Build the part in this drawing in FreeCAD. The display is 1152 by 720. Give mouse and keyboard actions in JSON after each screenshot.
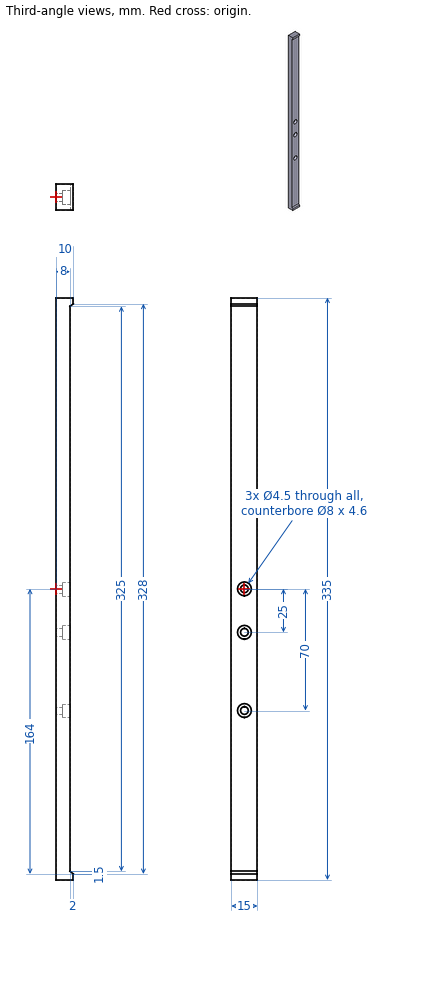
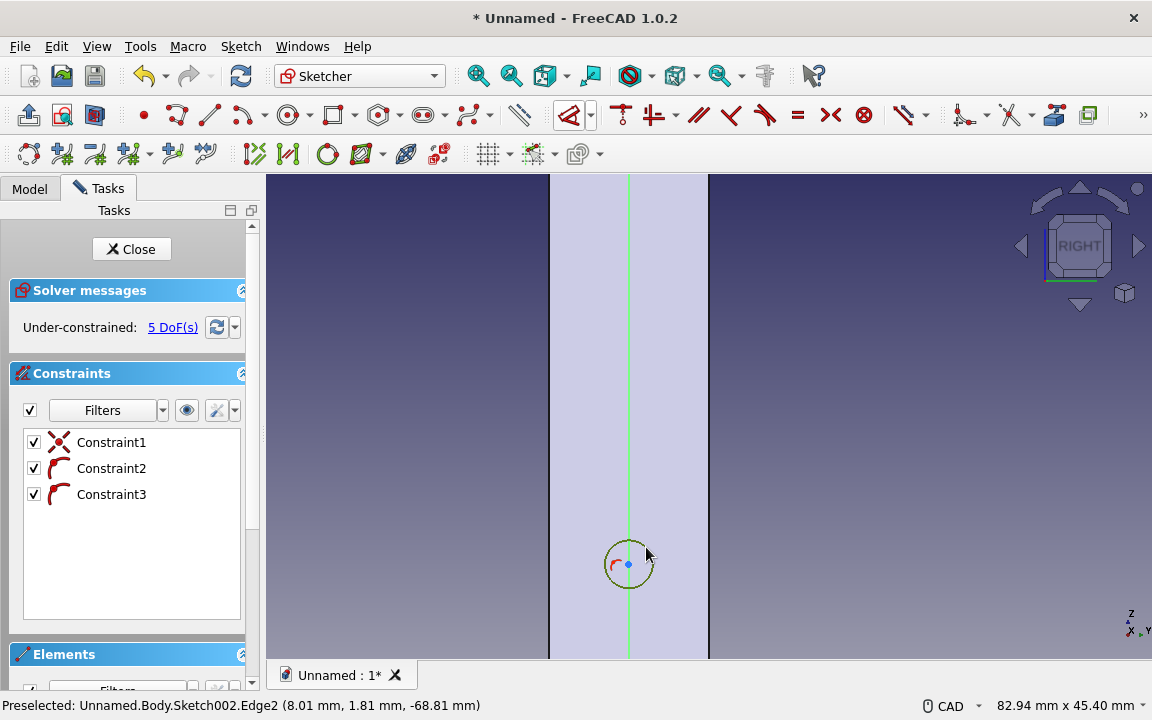
{"action": "scroll", "coordinate": [647, 549], "scroll_direction": "down", "scroll_amount": 5}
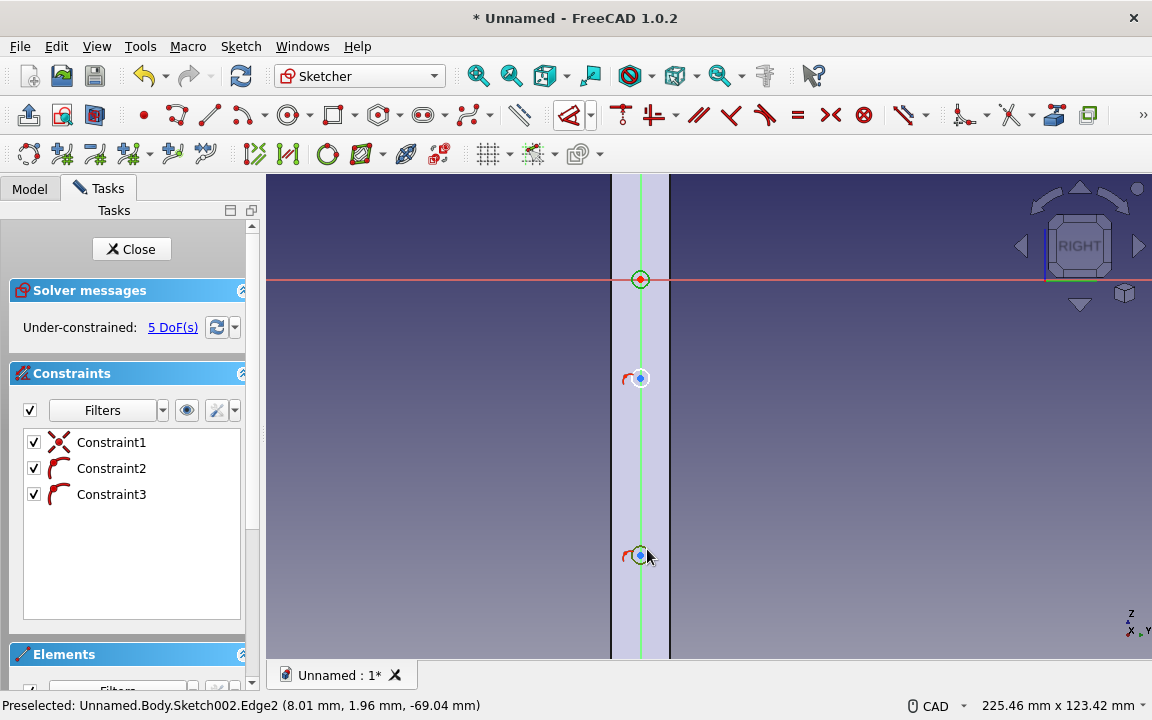
{"action": "scroll", "coordinate": [647, 372], "scroll_direction": "up", "scroll_amount": 5}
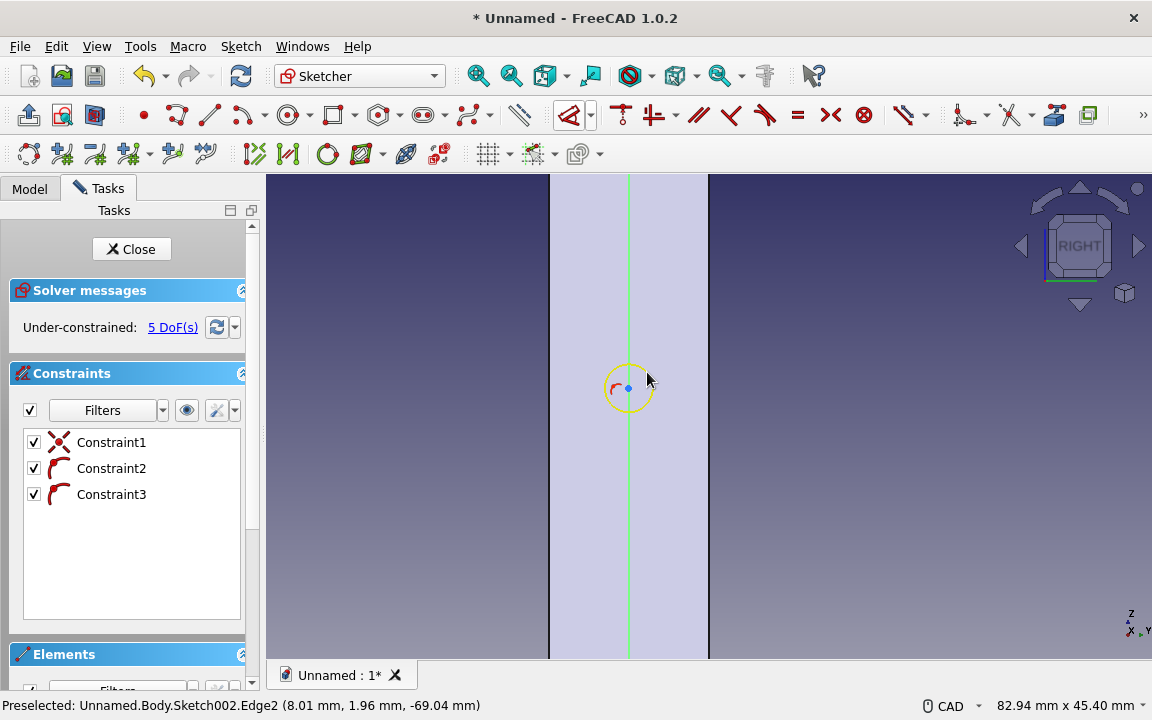
{"action": "left_click", "coordinate": [646, 371]}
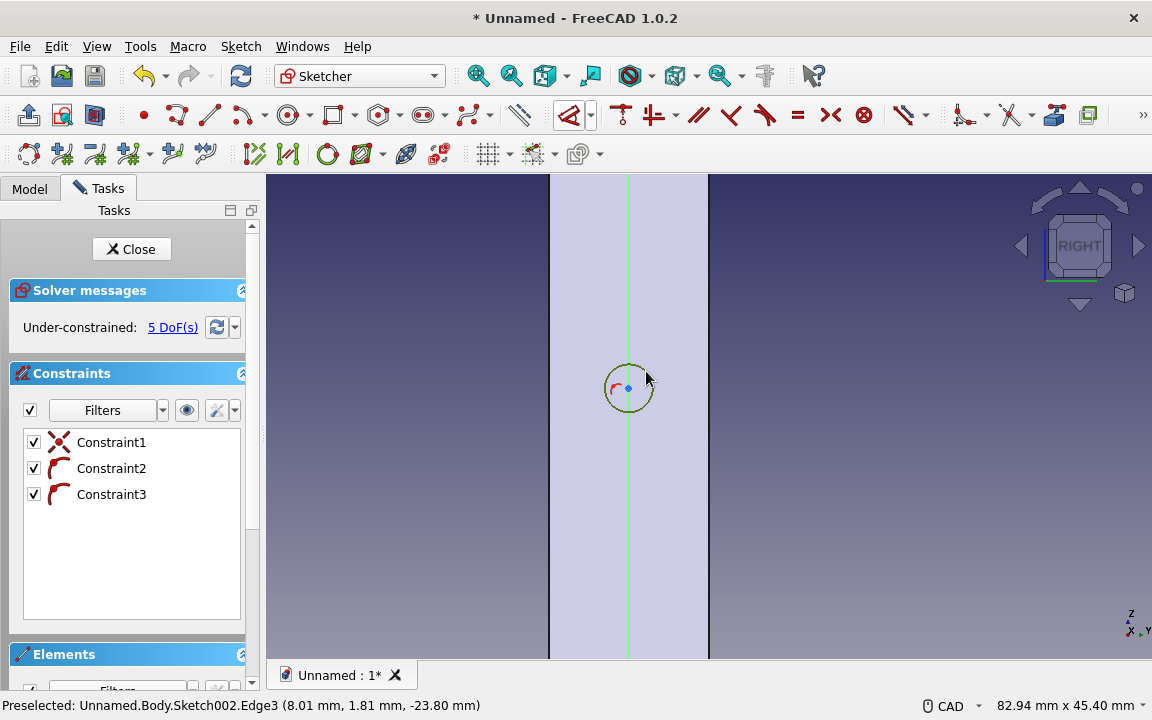
{"action": "left_click", "coordinate": [798, 116]}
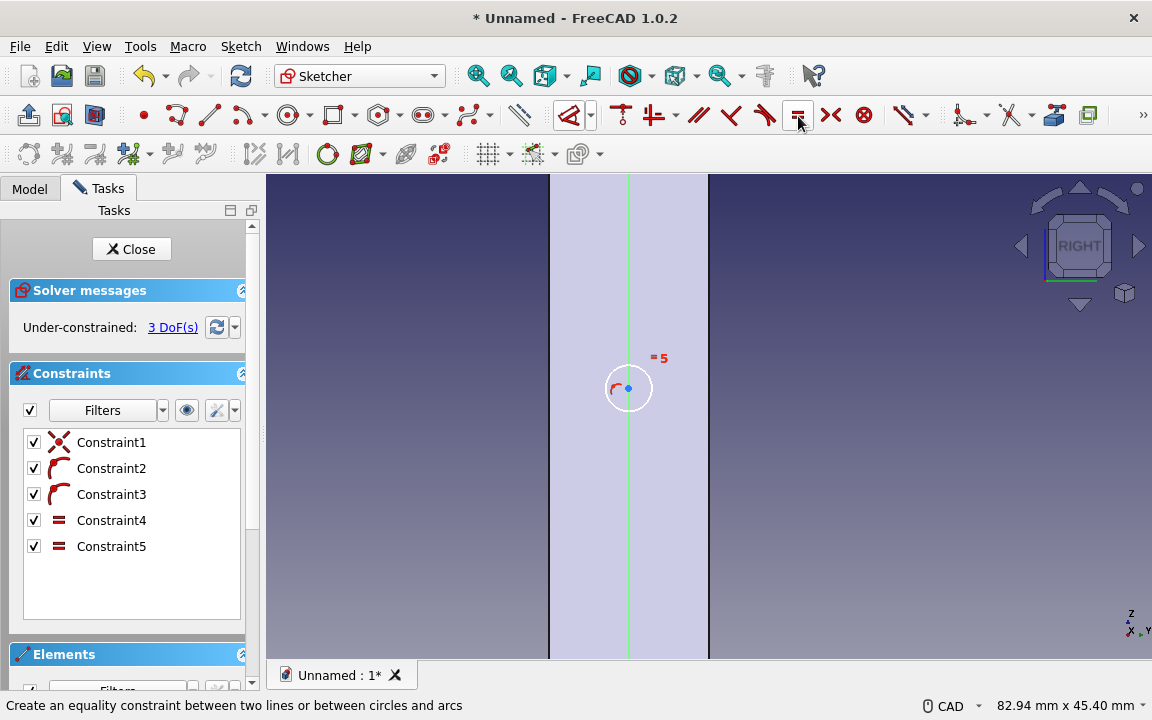
{"action": "scroll", "coordinate": [647, 371], "scroll_direction": "down", "scroll_amount": 5}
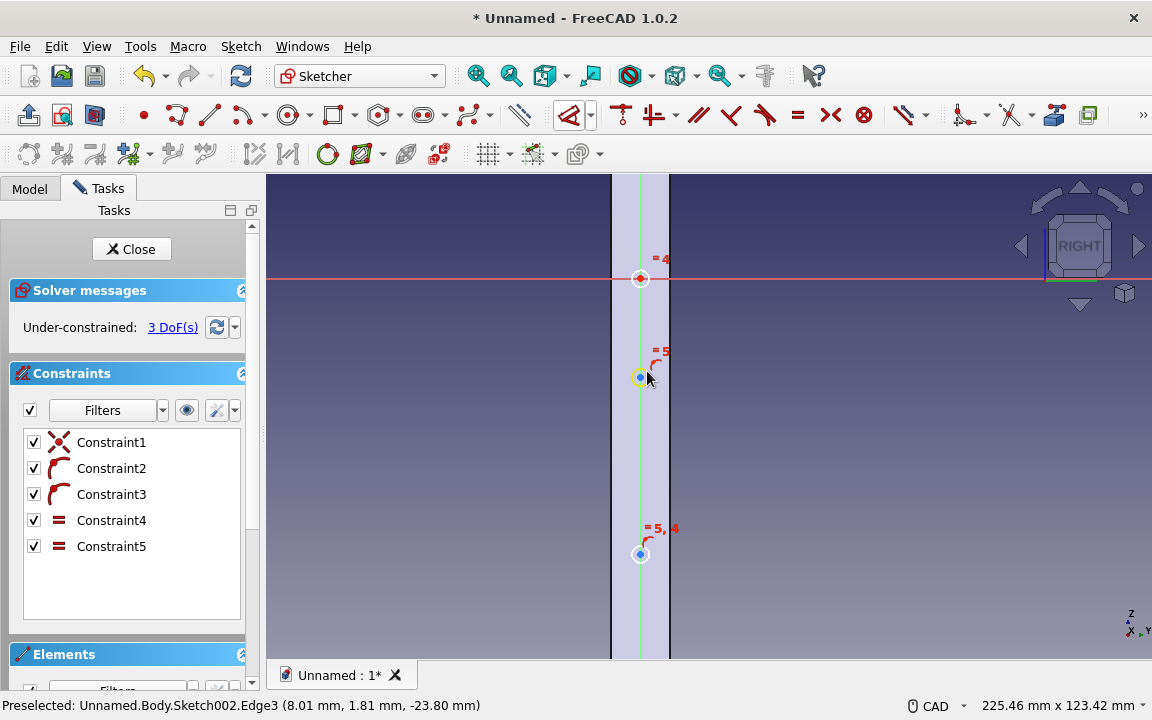
{"action": "scroll", "coordinate": [647, 273], "scroll_direction": "up", "scroll_amount": 5}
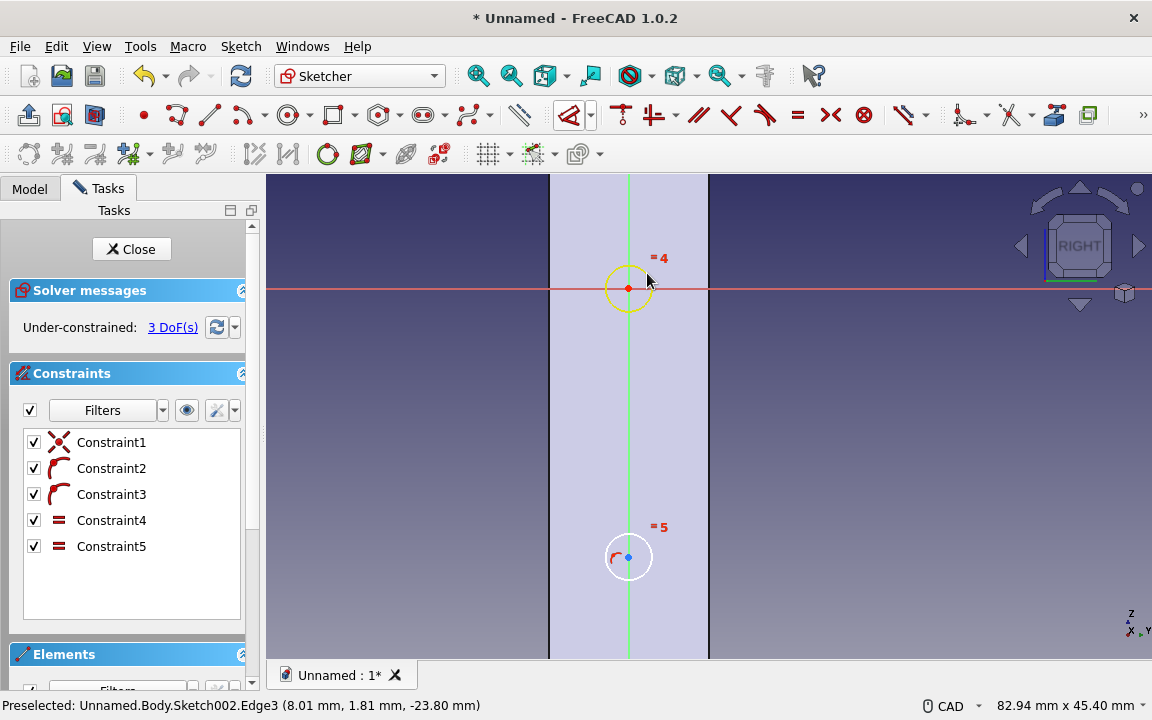
{"action": "left_click", "coordinate": [645, 272]}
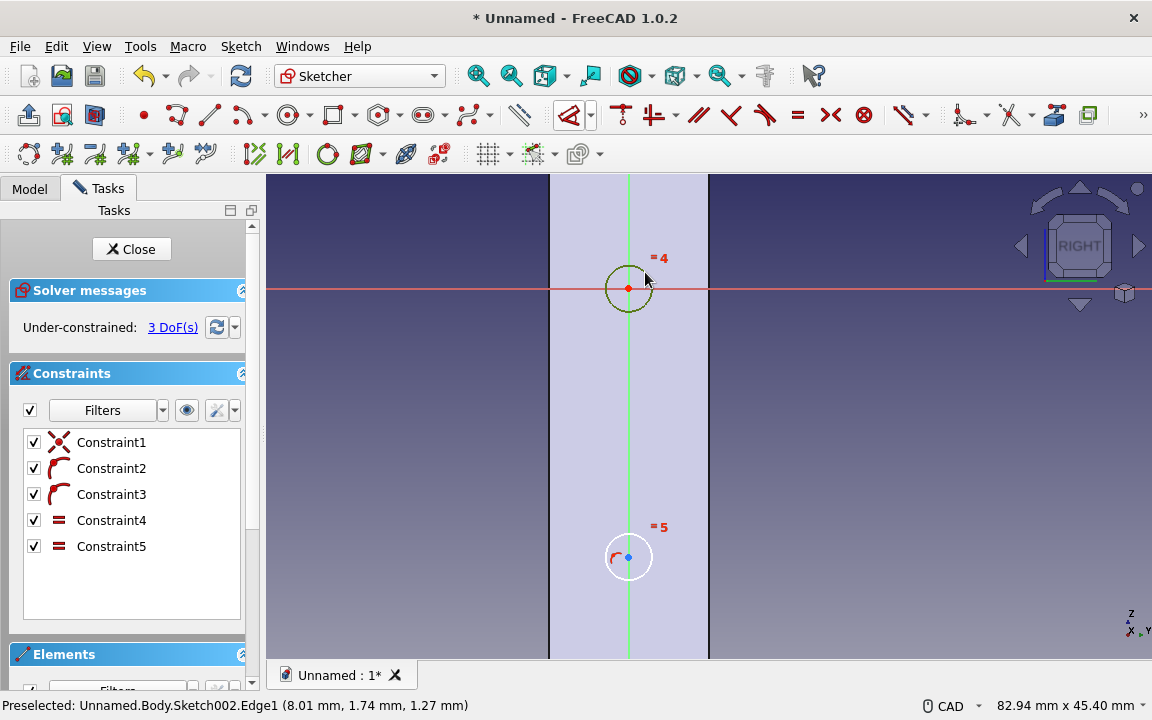
{"action": "left_click", "coordinate": [590, 116]}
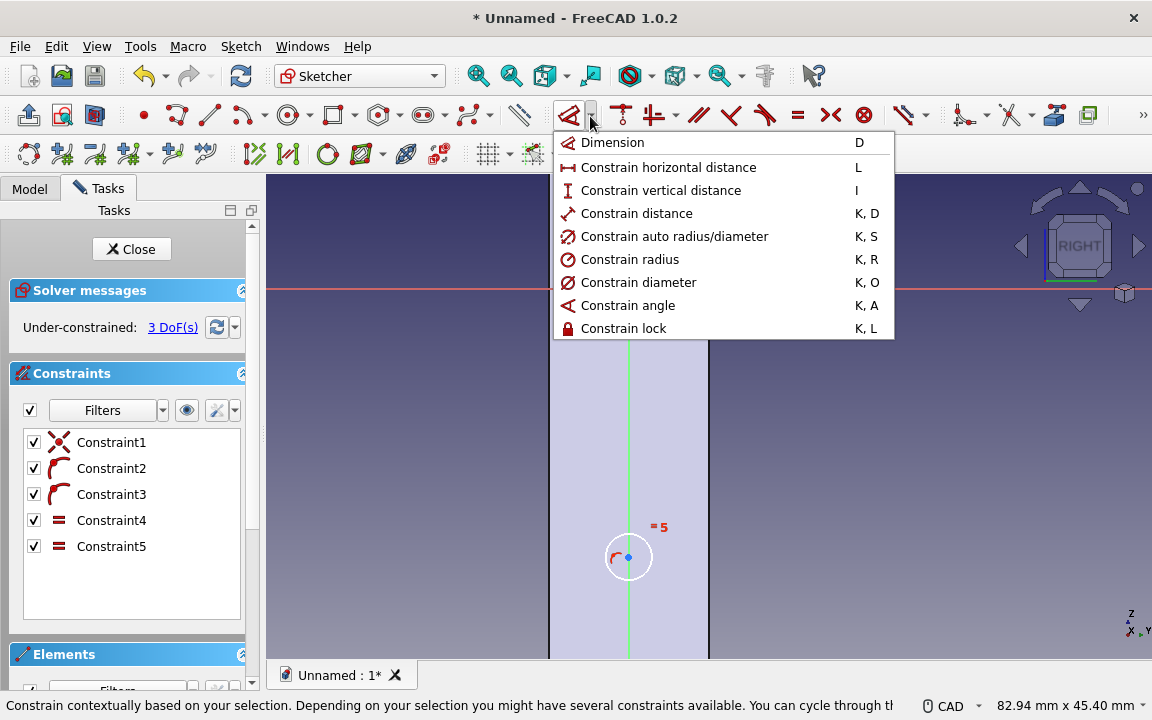
{"action": "left_click", "coordinate": [724, 282]}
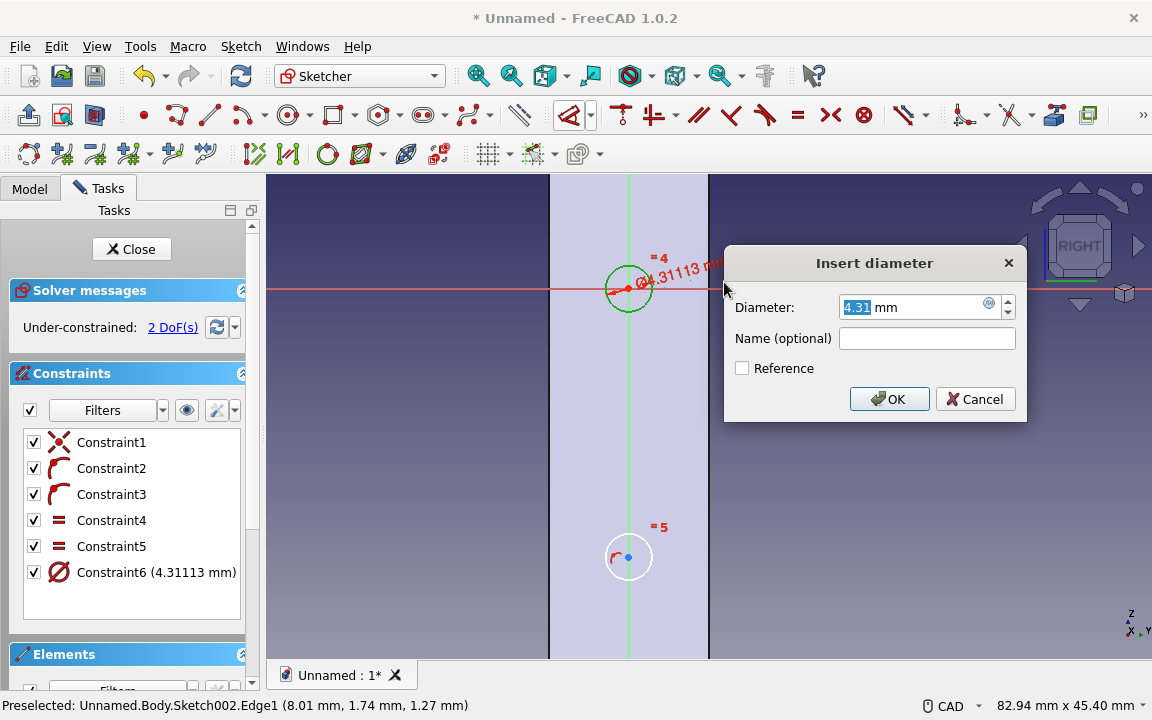
{"action": "type", "text": "4.5"}
{"action": "key", "text": "Return"}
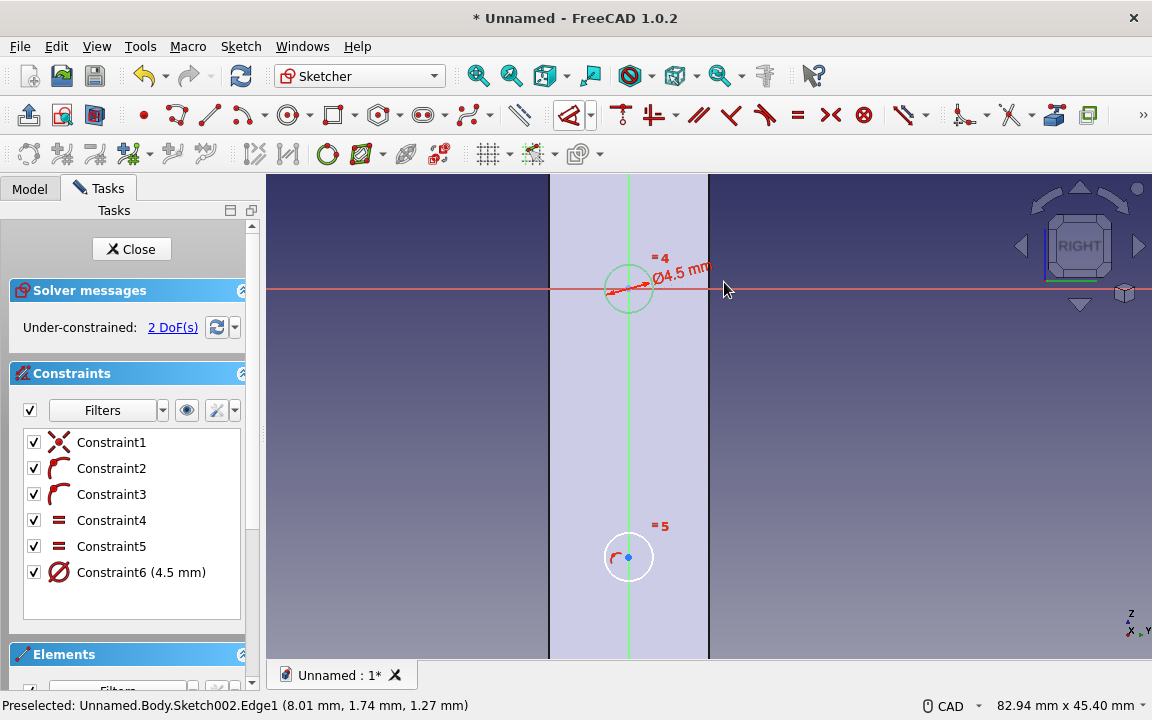
{"action": "scroll", "coordinate": [647, 273], "scroll_direction": "down", "scroll_amount": 5}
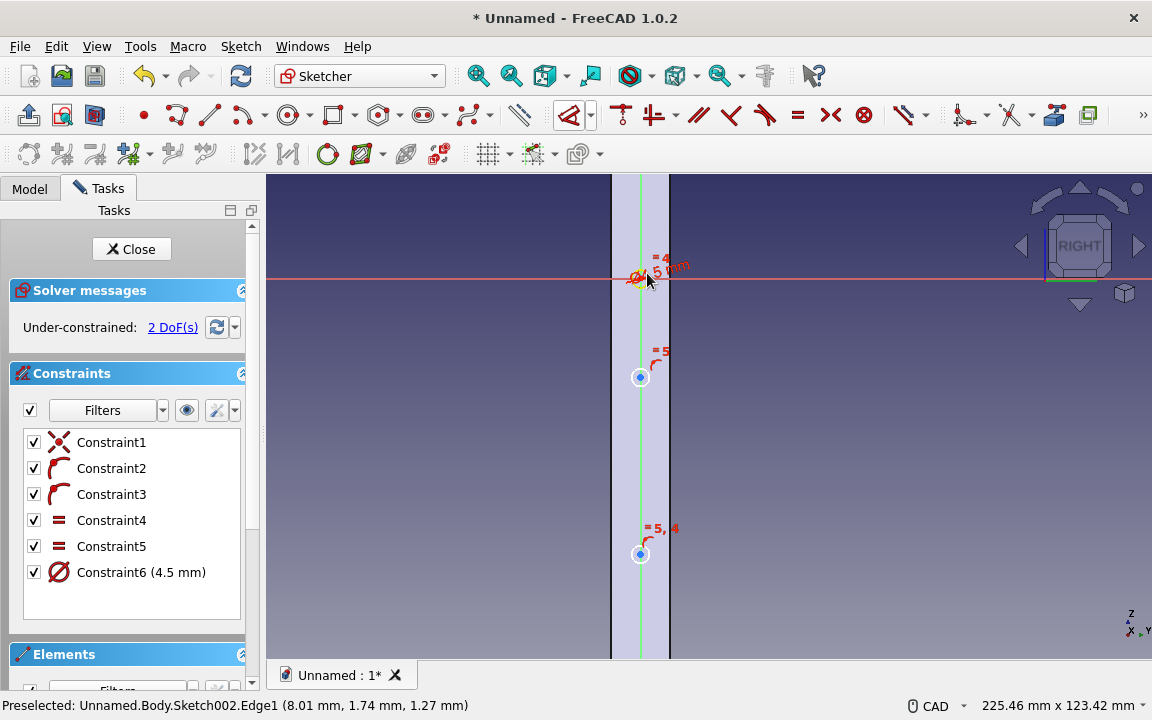
{"action": "left_click", "coordinate": [641, 554]}